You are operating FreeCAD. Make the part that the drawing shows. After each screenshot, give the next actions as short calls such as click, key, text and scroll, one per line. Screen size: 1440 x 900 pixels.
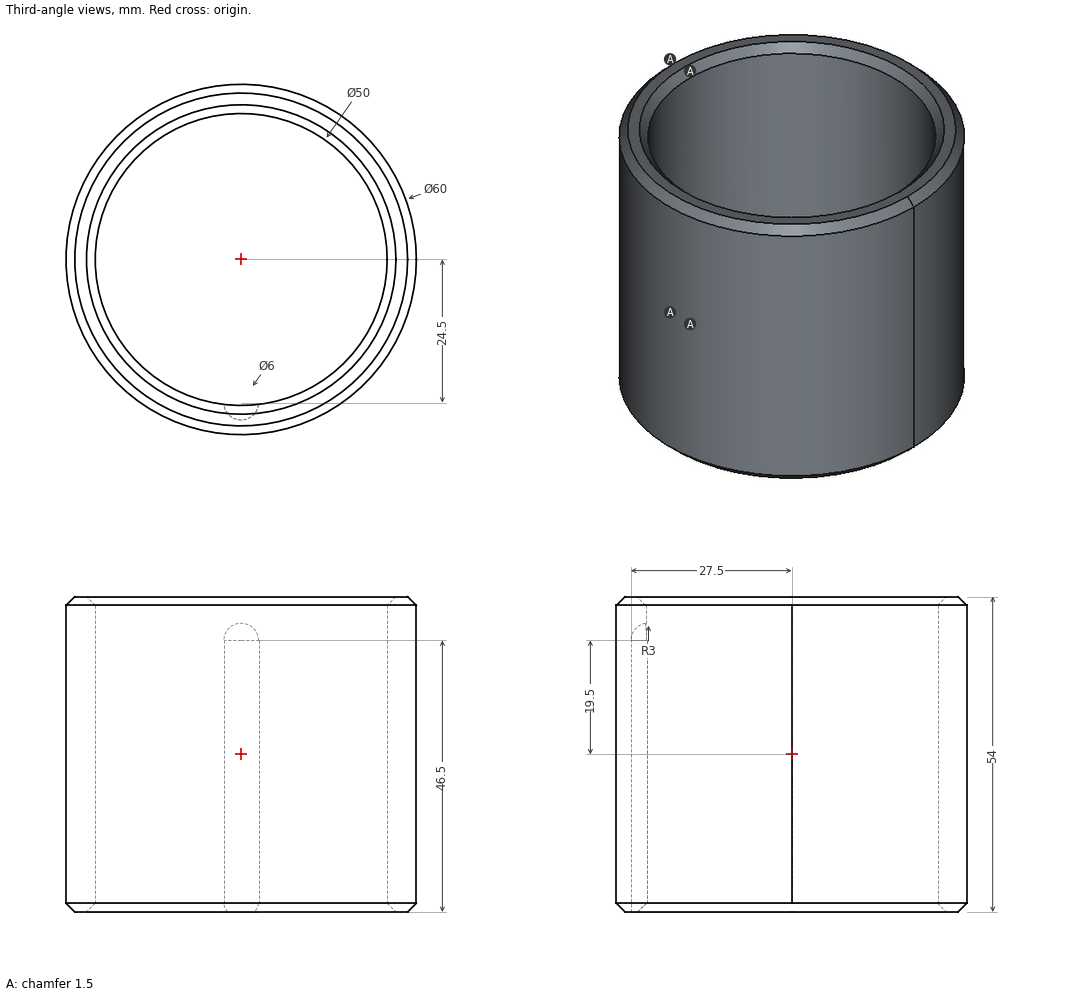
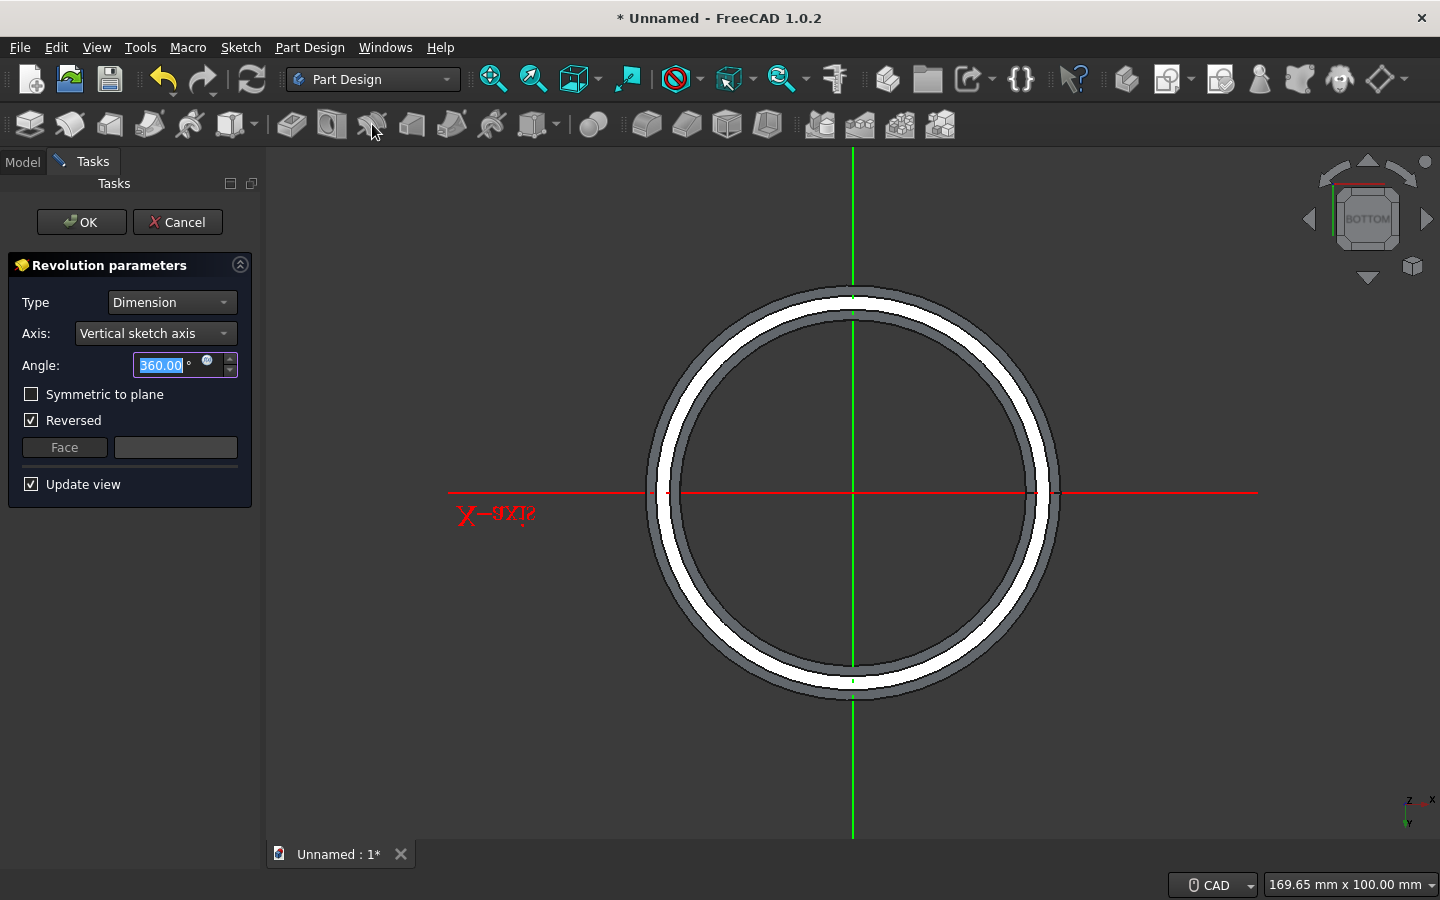
click(156, 334)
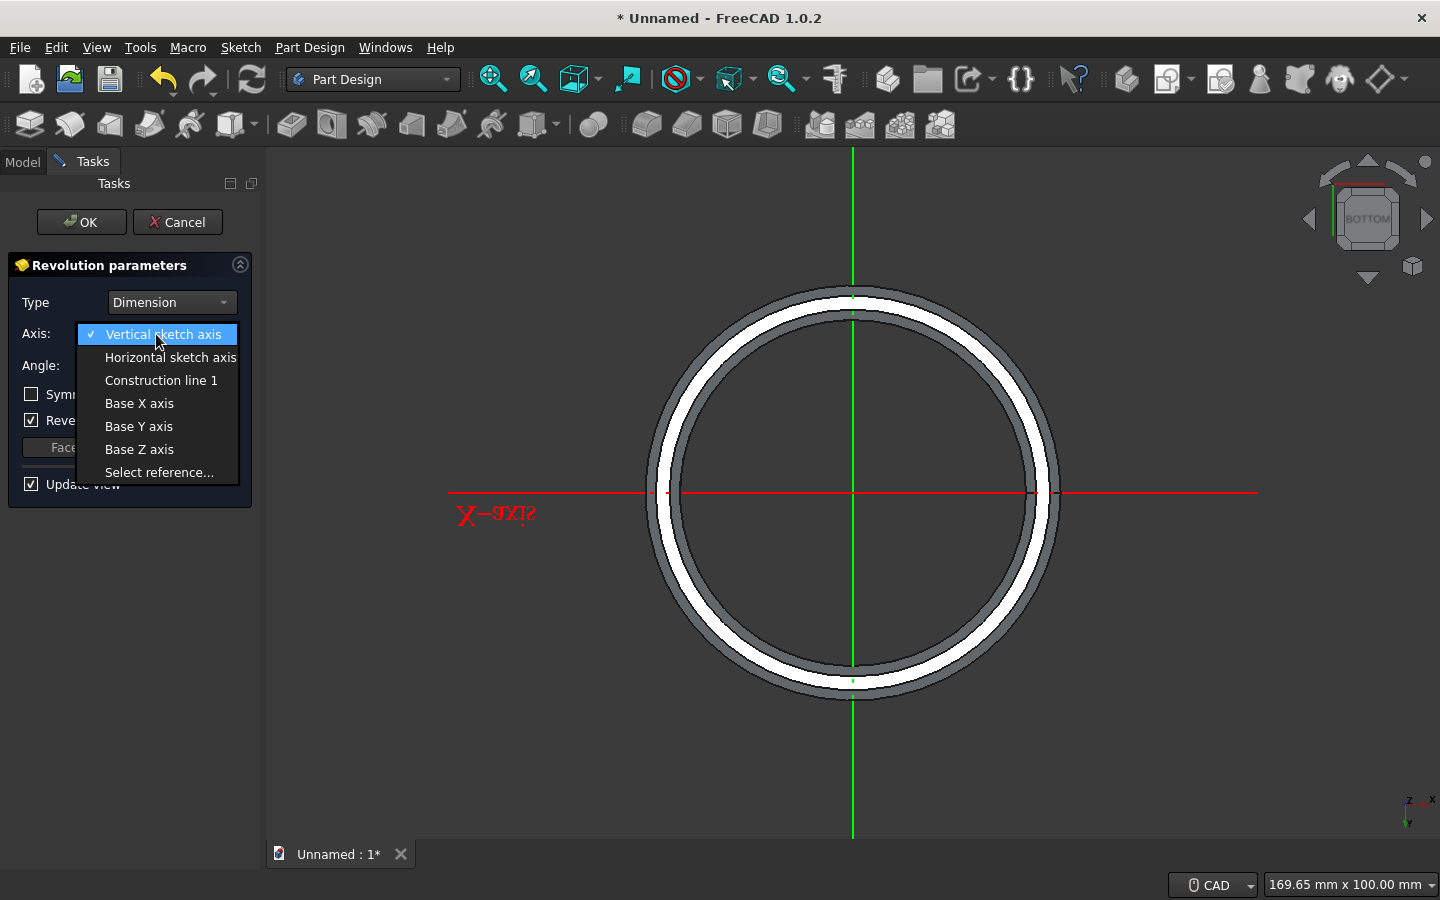
click(156, 380)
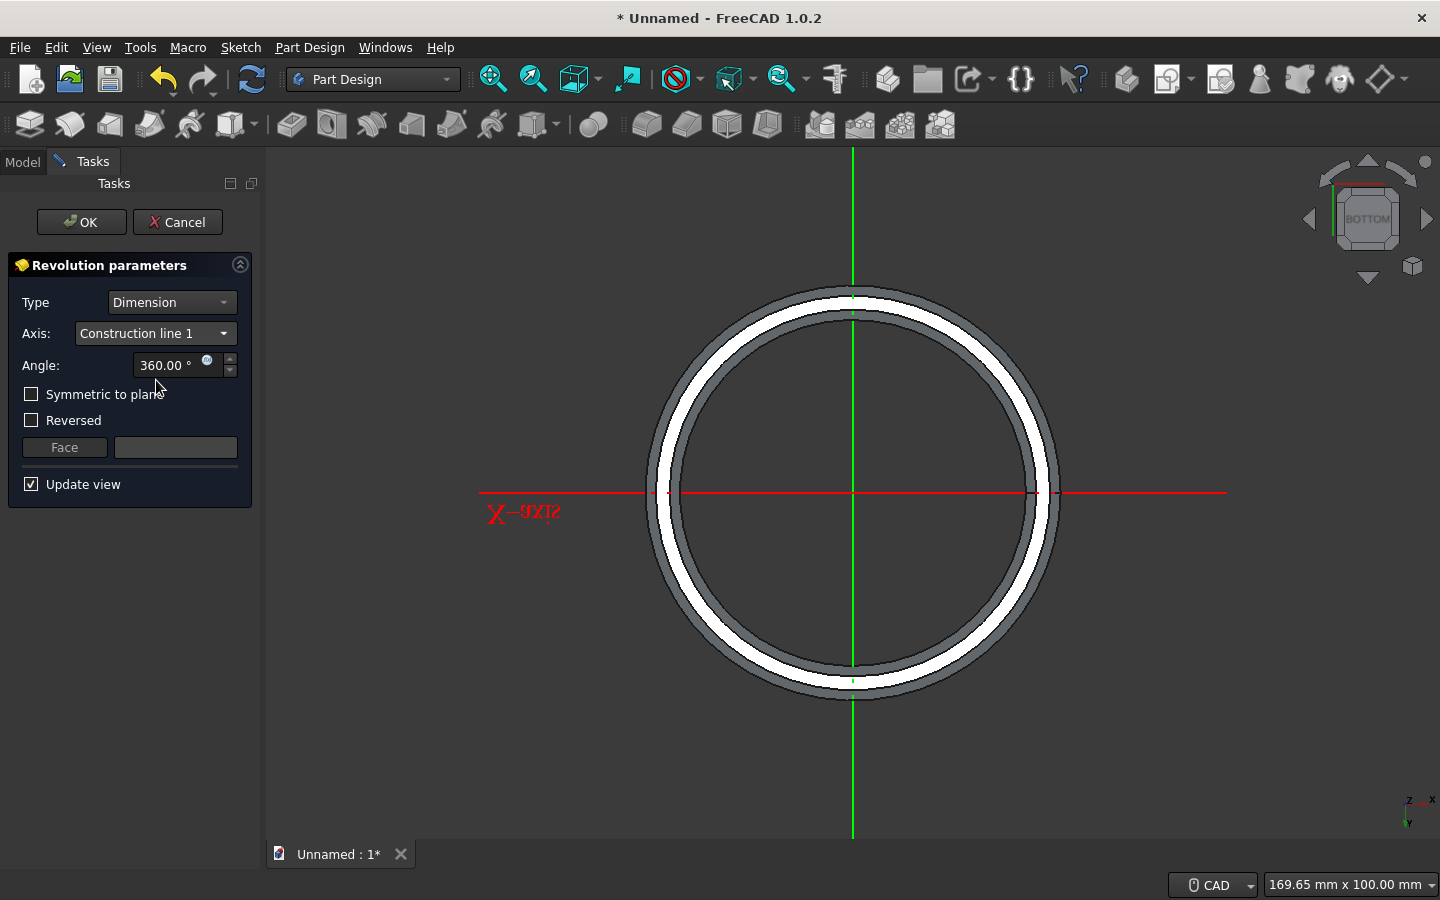
click(82, 222)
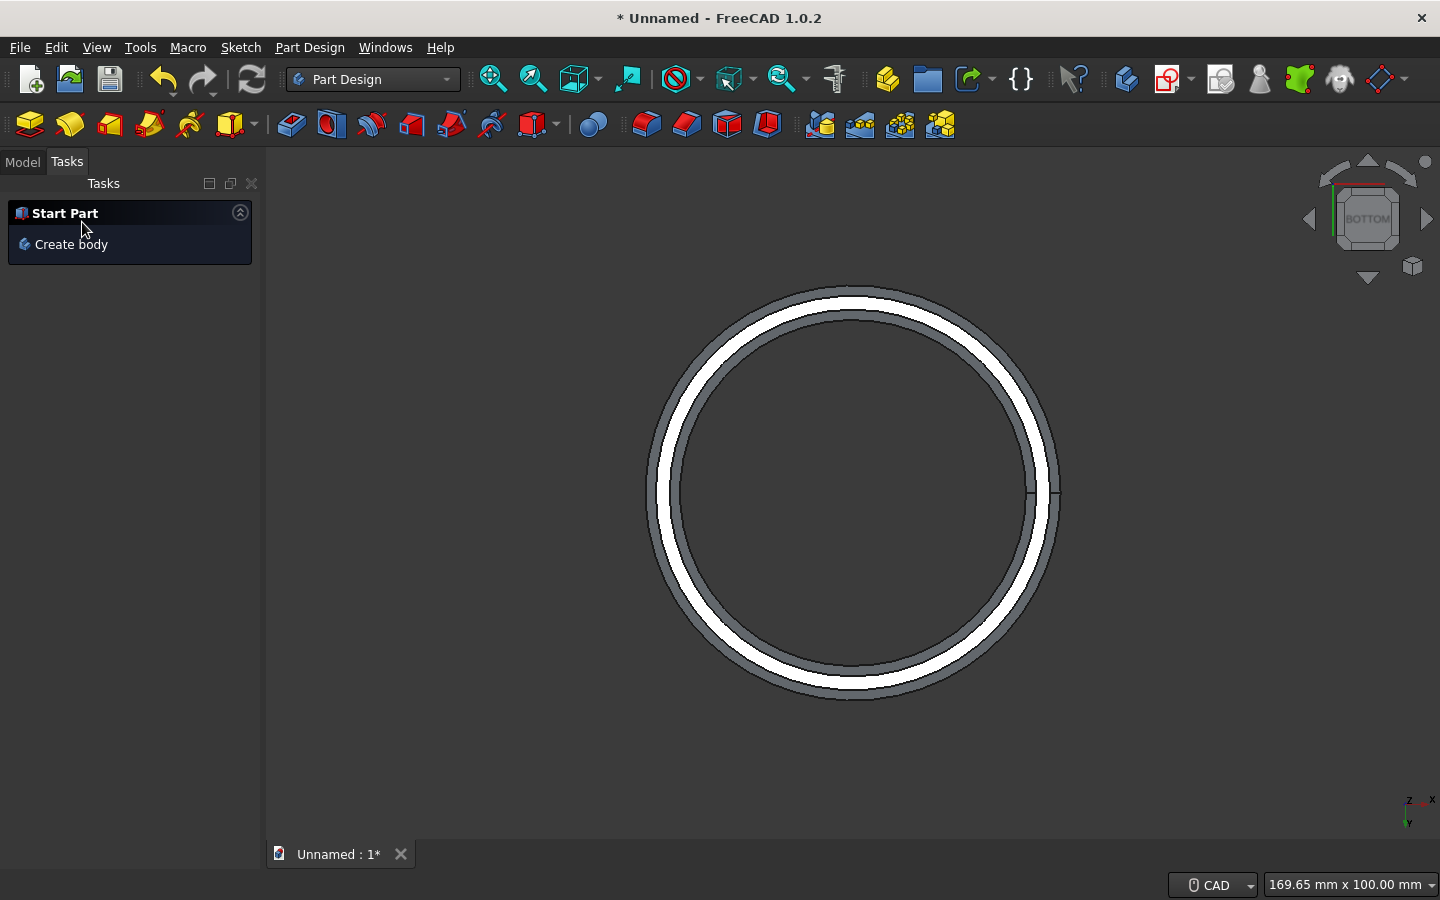
click(23, 161)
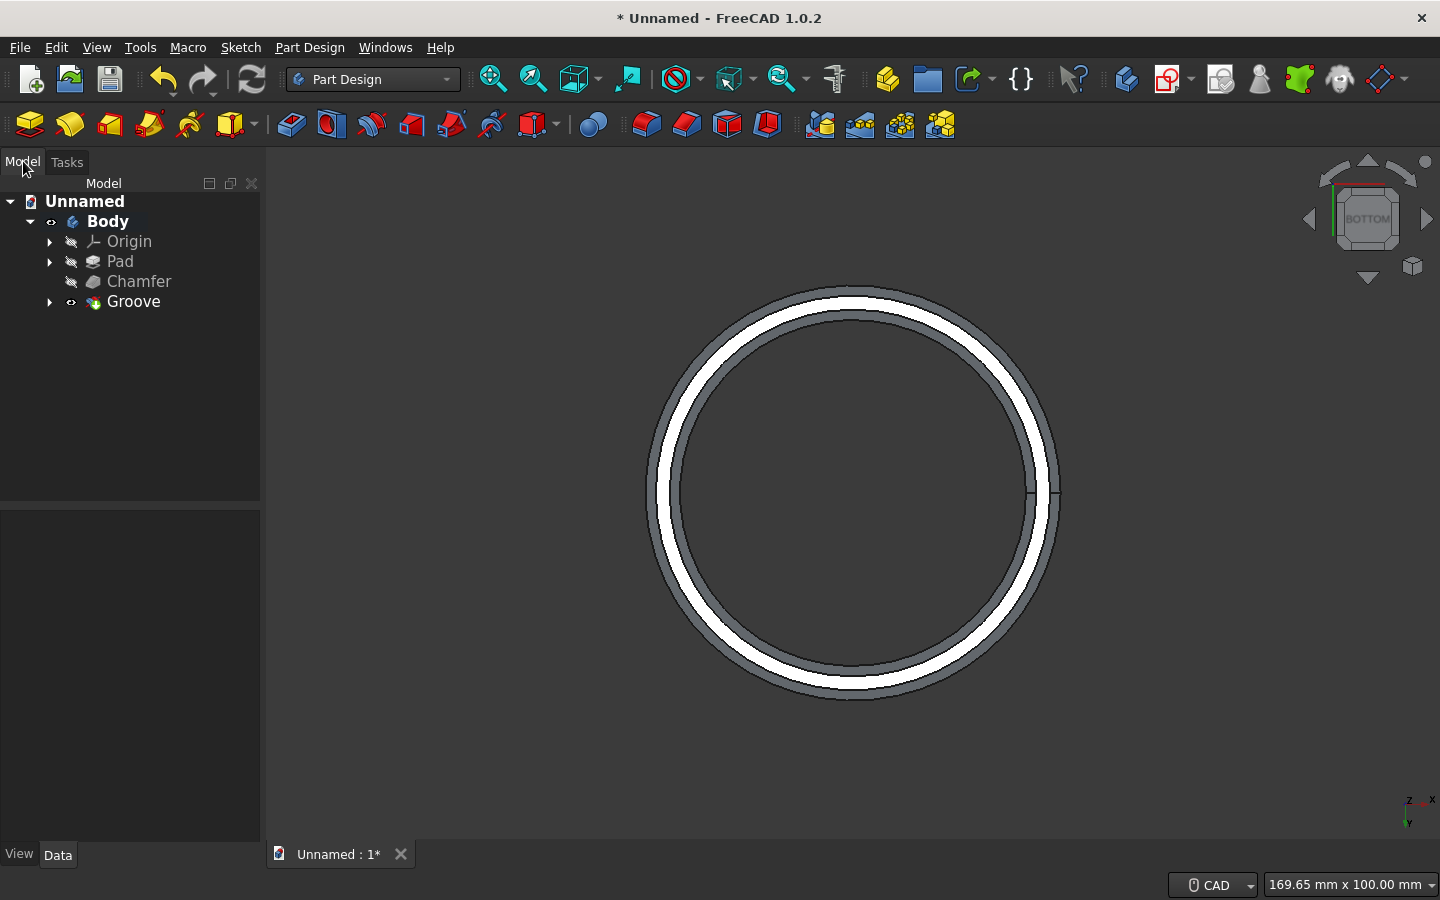
click(50, 242)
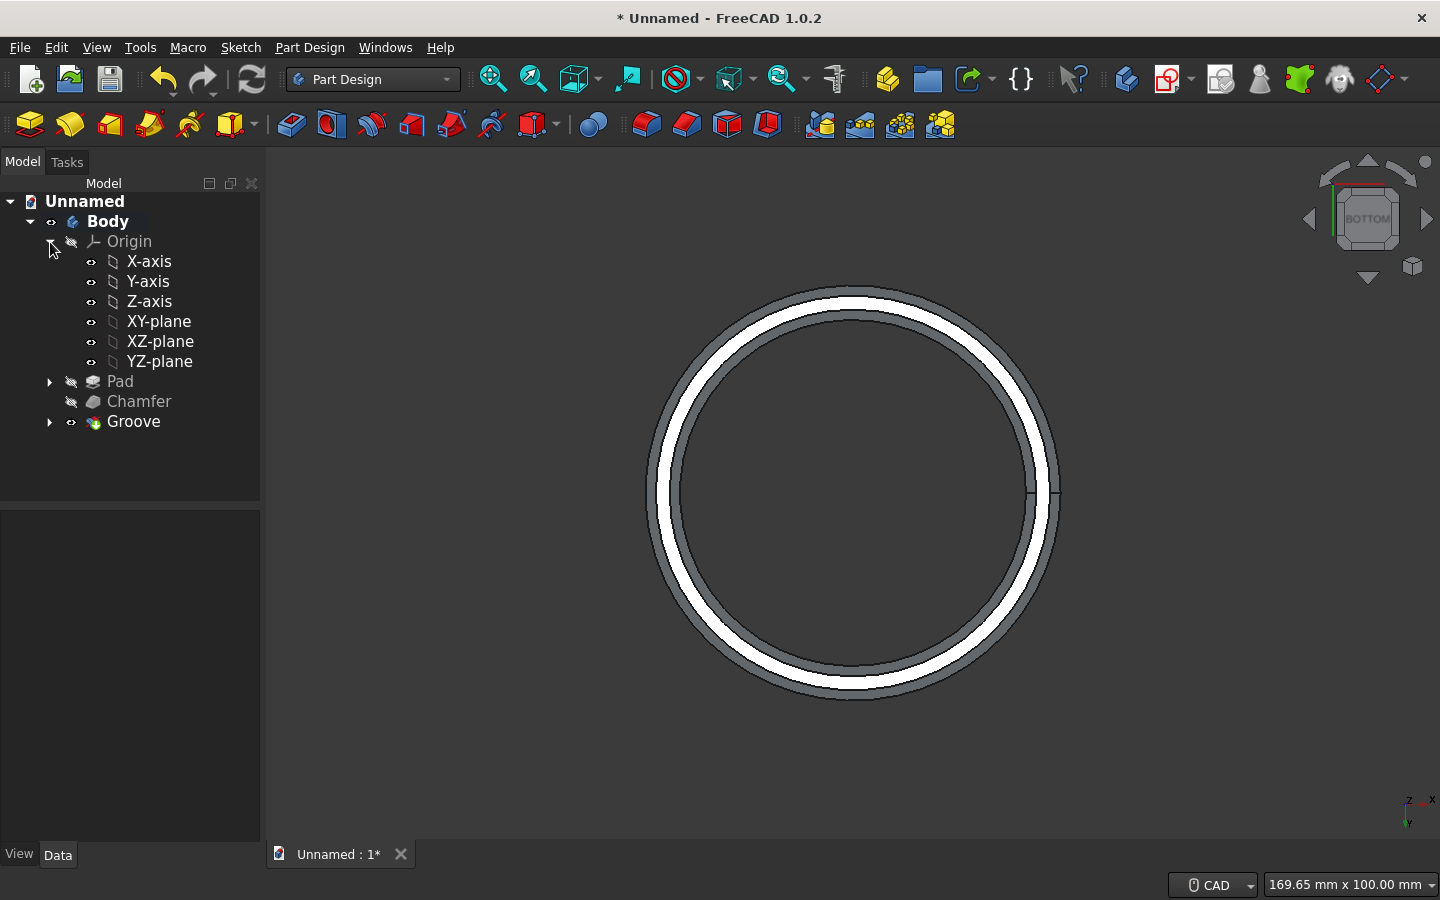
click(136, 322)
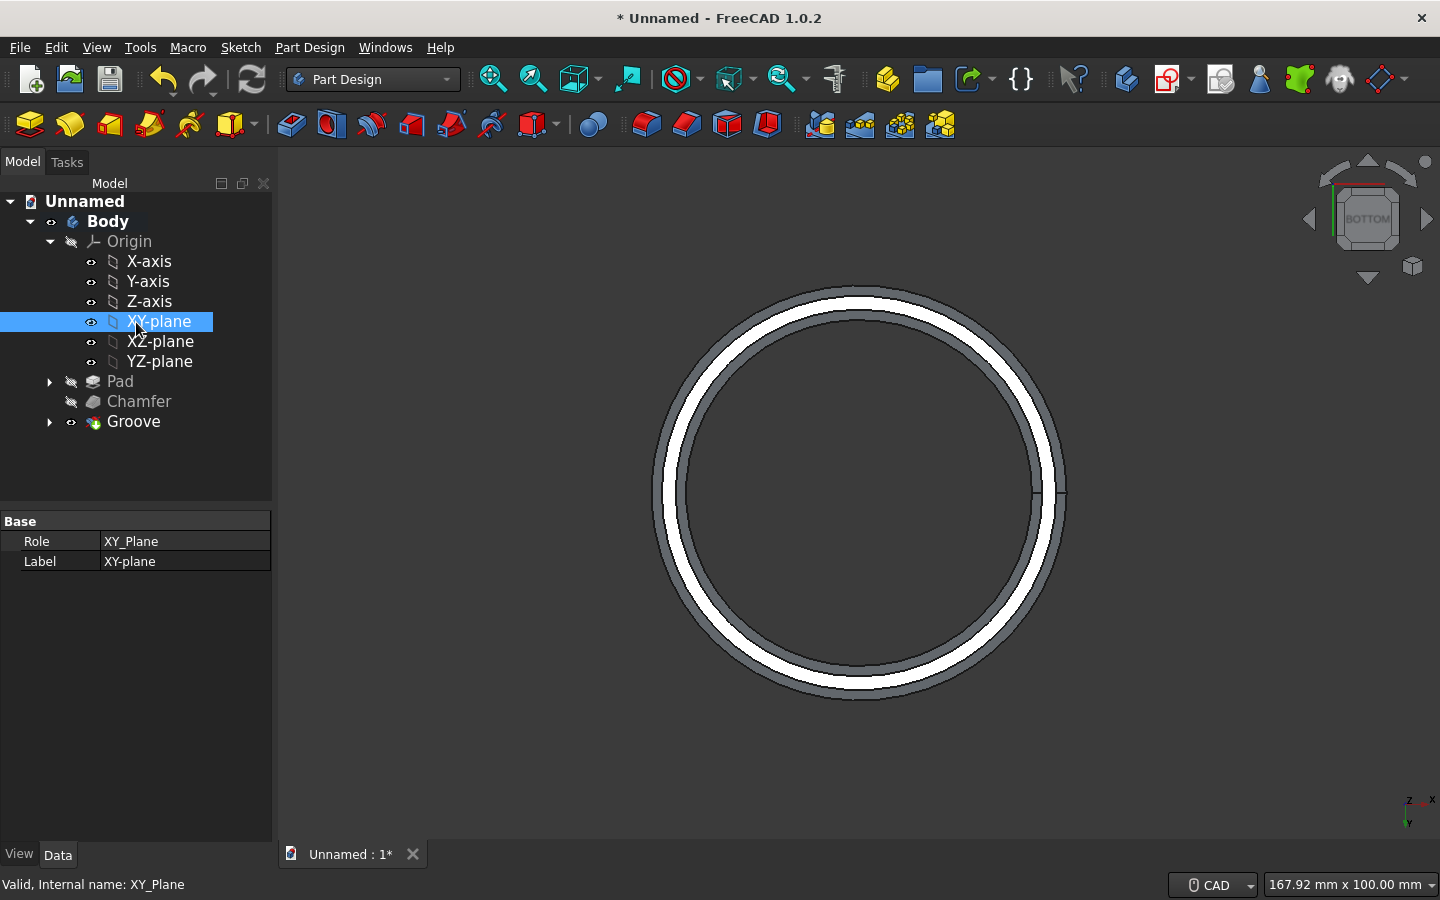
click(1380, 80)